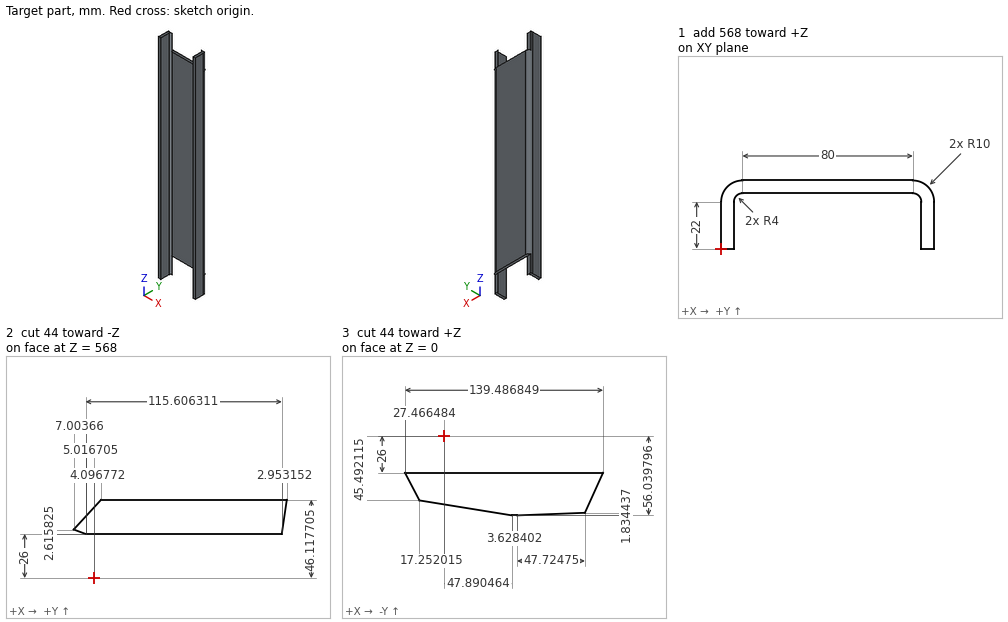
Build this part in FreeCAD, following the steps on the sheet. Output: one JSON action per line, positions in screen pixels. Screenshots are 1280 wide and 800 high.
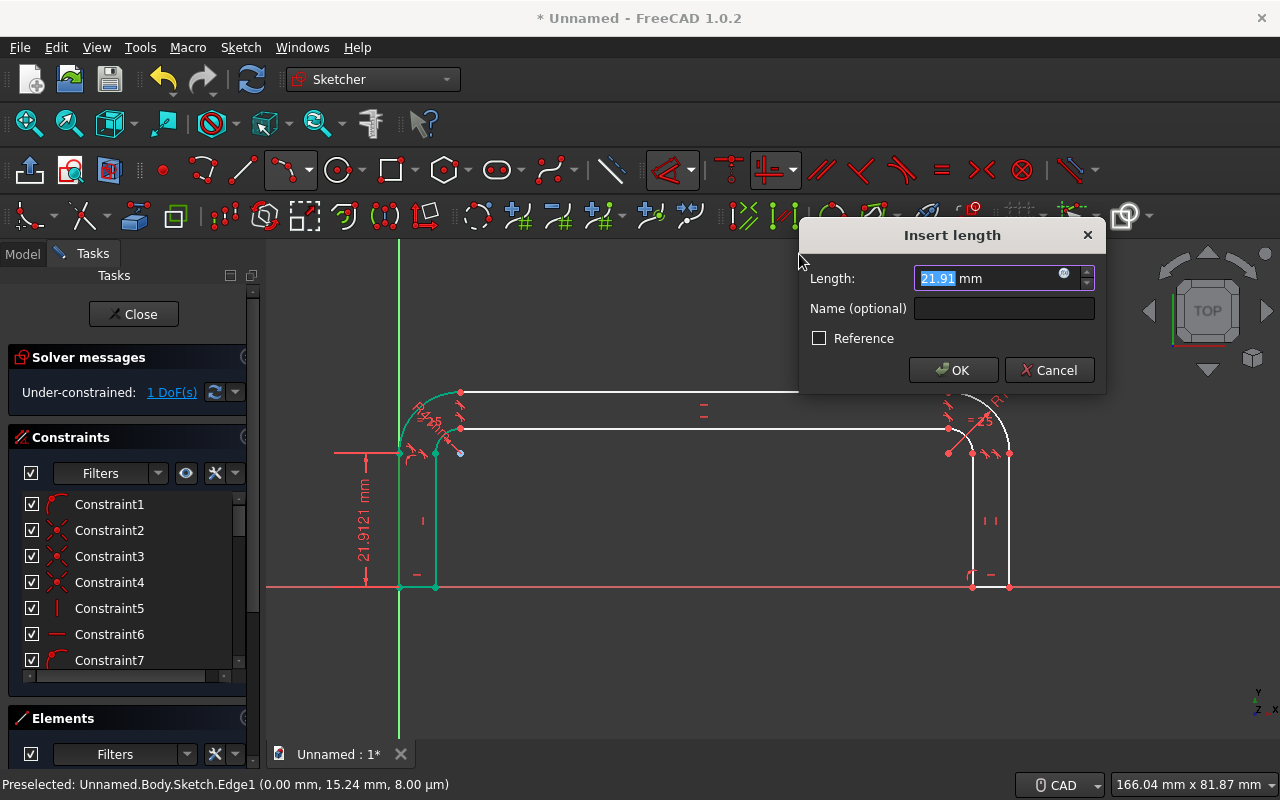
{"action": "type", "text": "22"}
{"action": "key", "text": "Return"}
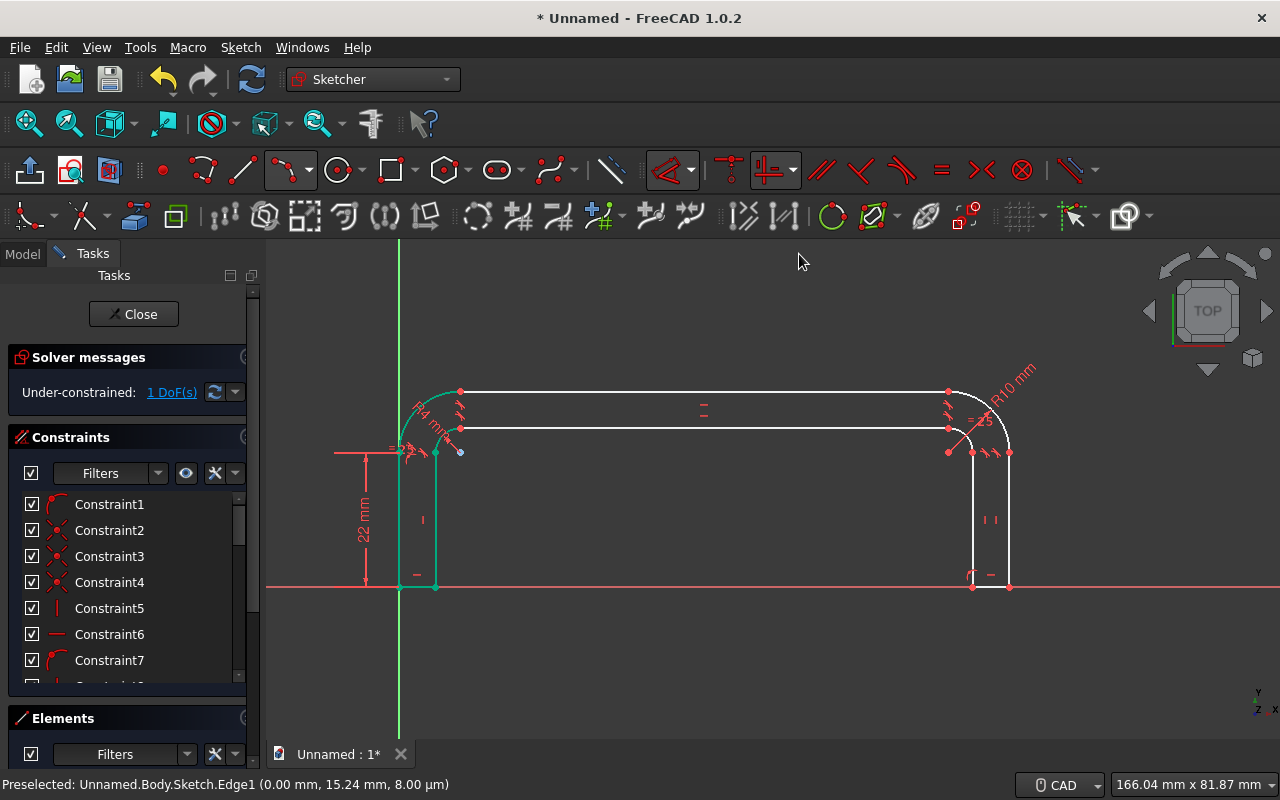
{"action": "left_click", "coordinate": [607, 428]}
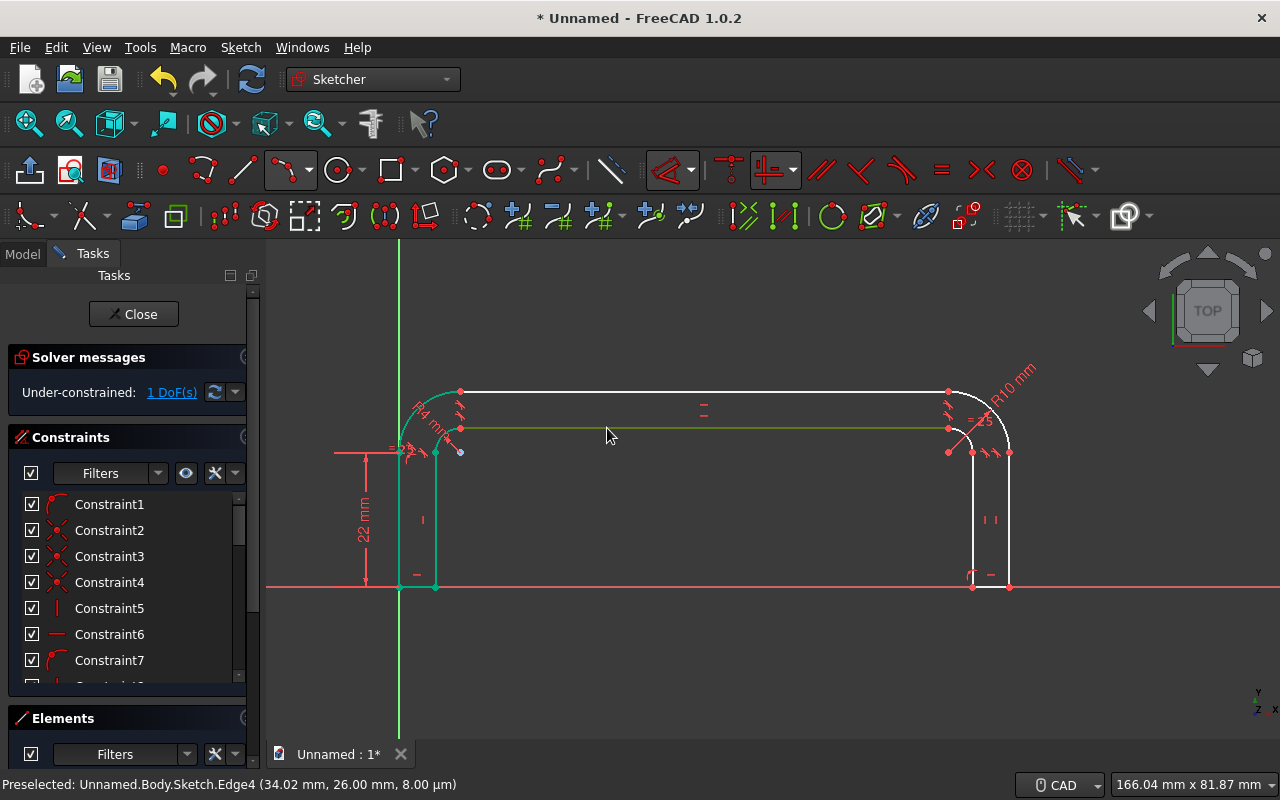
{"action": "left_click", "coordinate": [694, 170]}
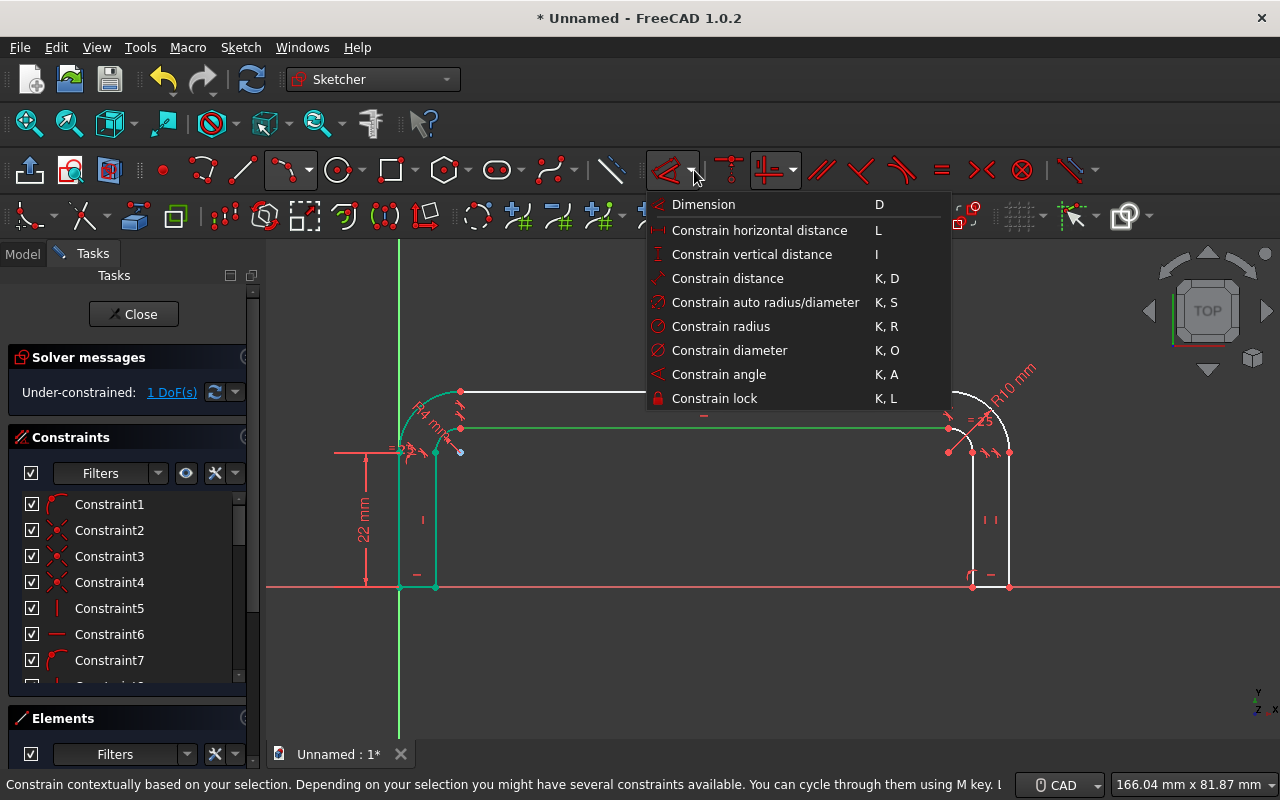
{"action": "left_click", "coordinate": [799, 230]}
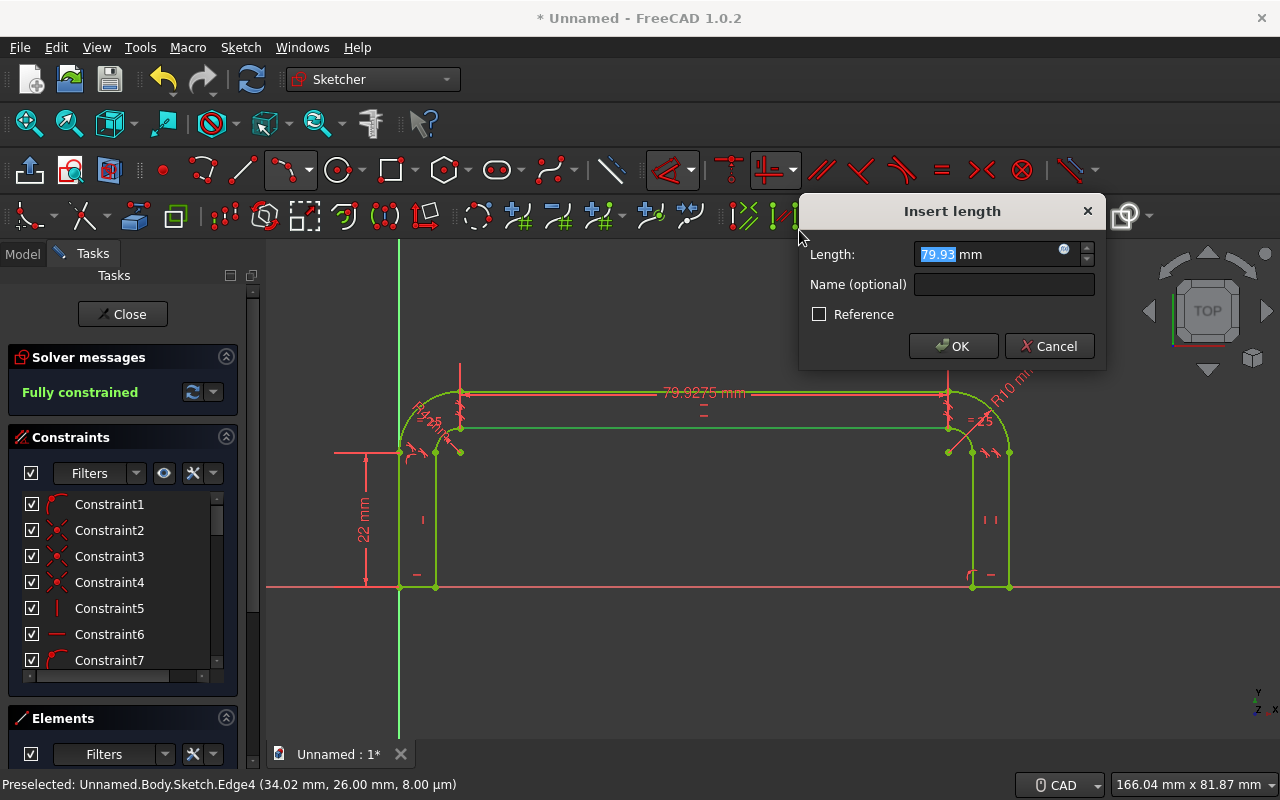
{"action": "type", "text": "80"}
{"action": "key", "text": "Return"}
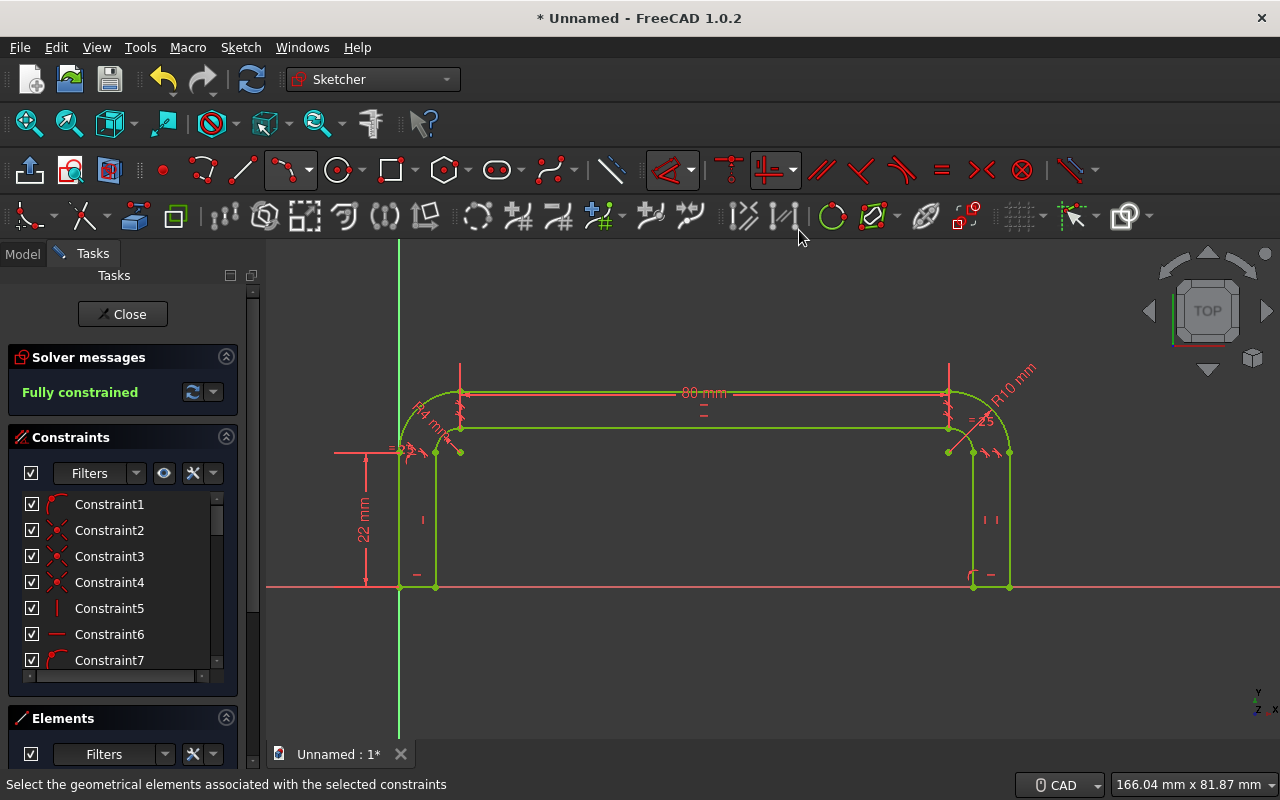
{"action": "left_click", "coordinate": [123, 314]}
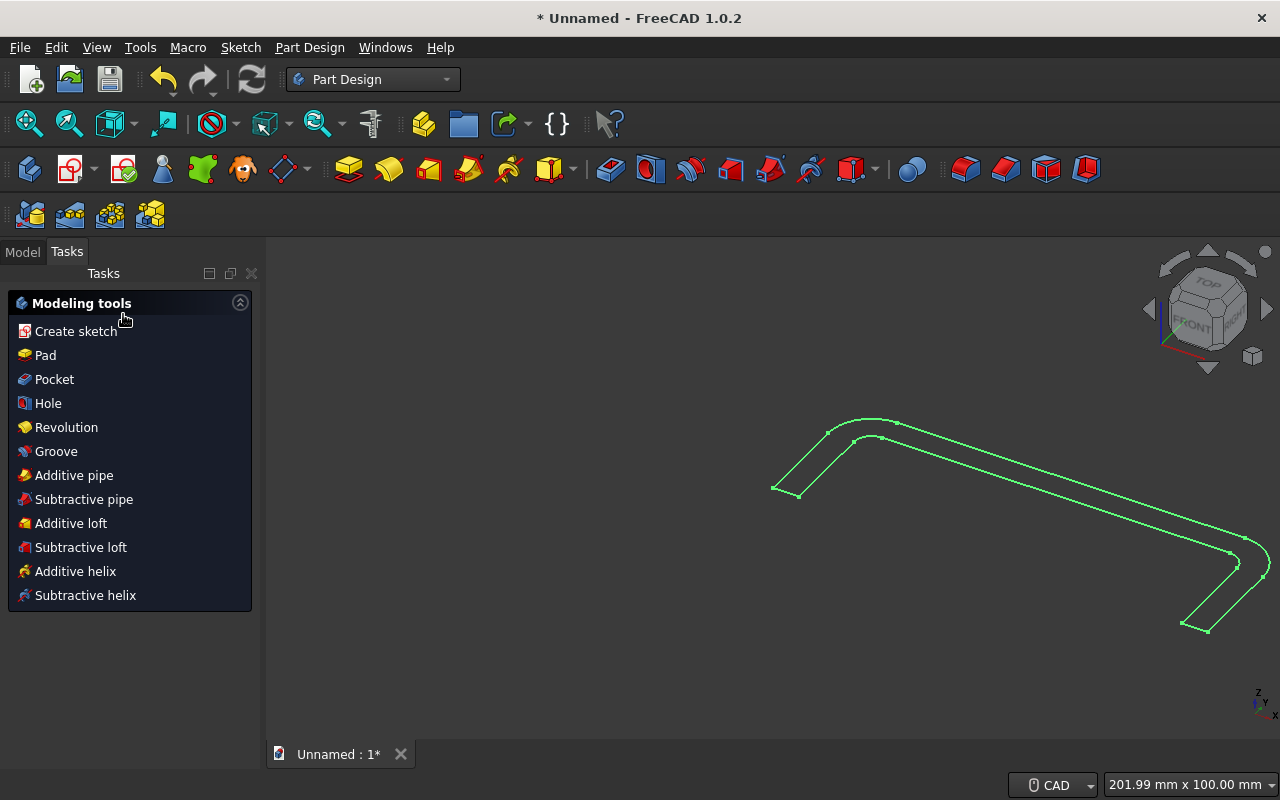
{"action": "left_click", "coordinate": [350, 170]}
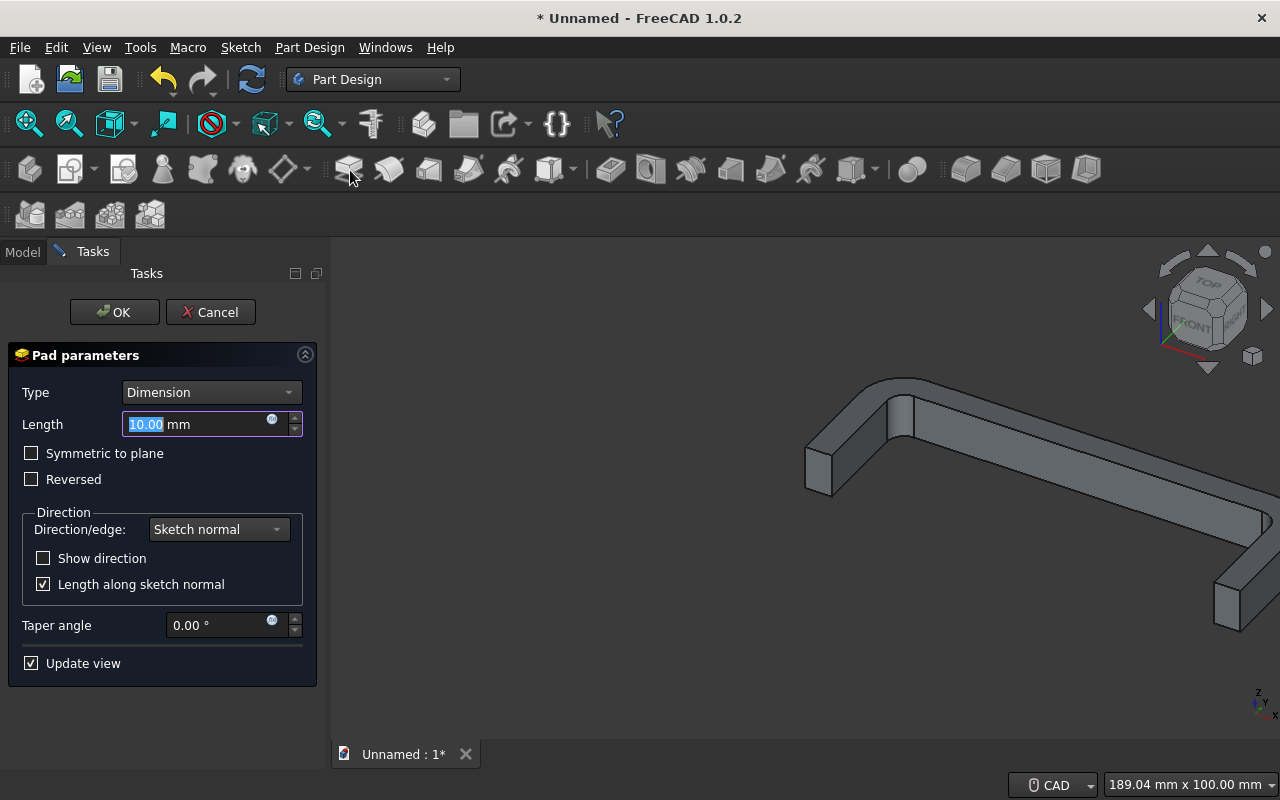
{"action": "type", "text": "568"}
{"action": "key", "text": "Tab"}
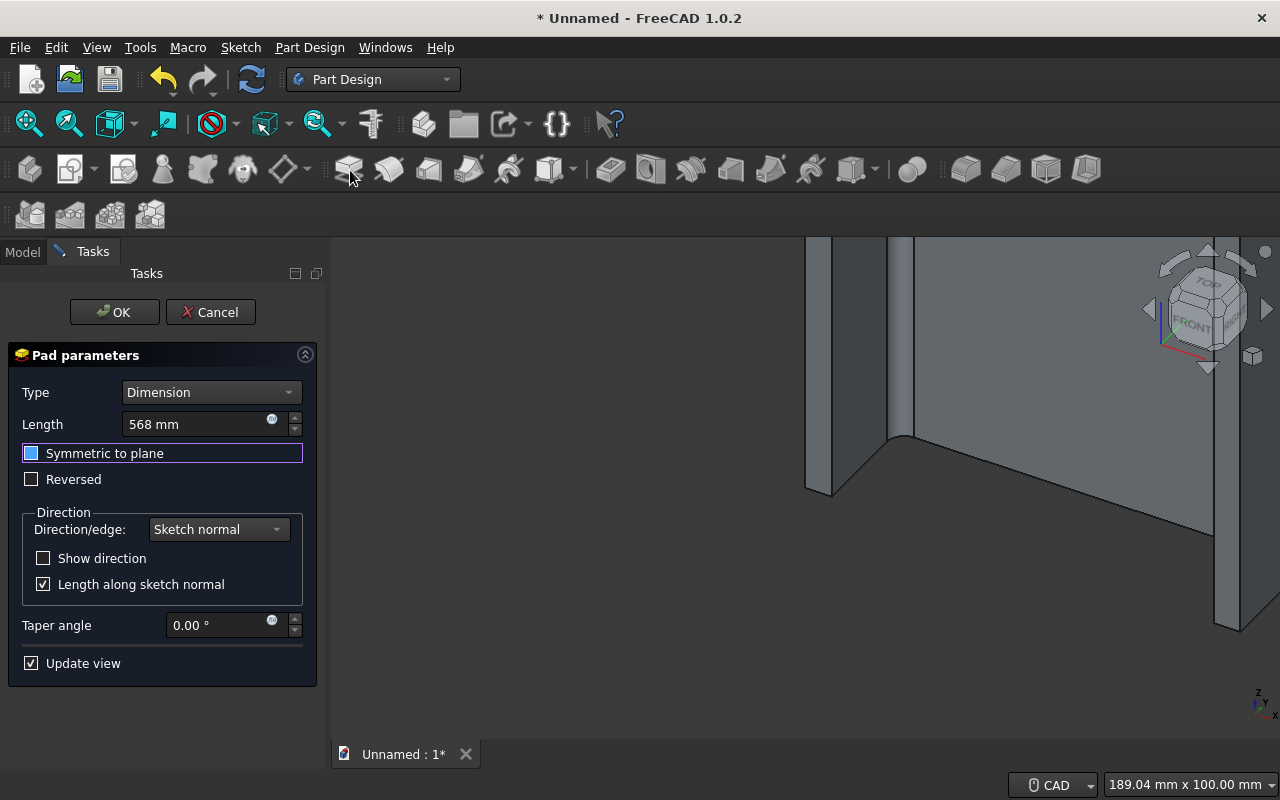
{"action": "left_click", "coordinate": [115, 312]}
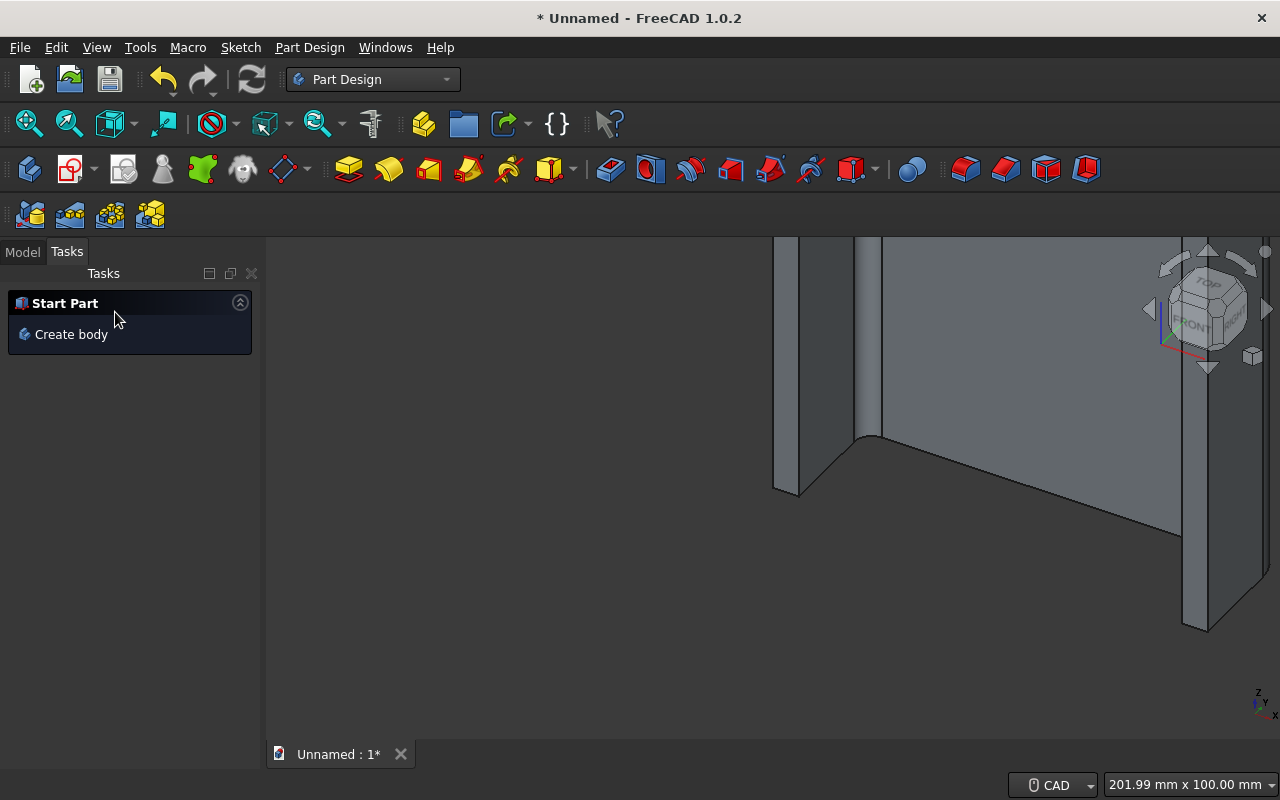
{"action": "left_click", "coordinate": [30, 124]}